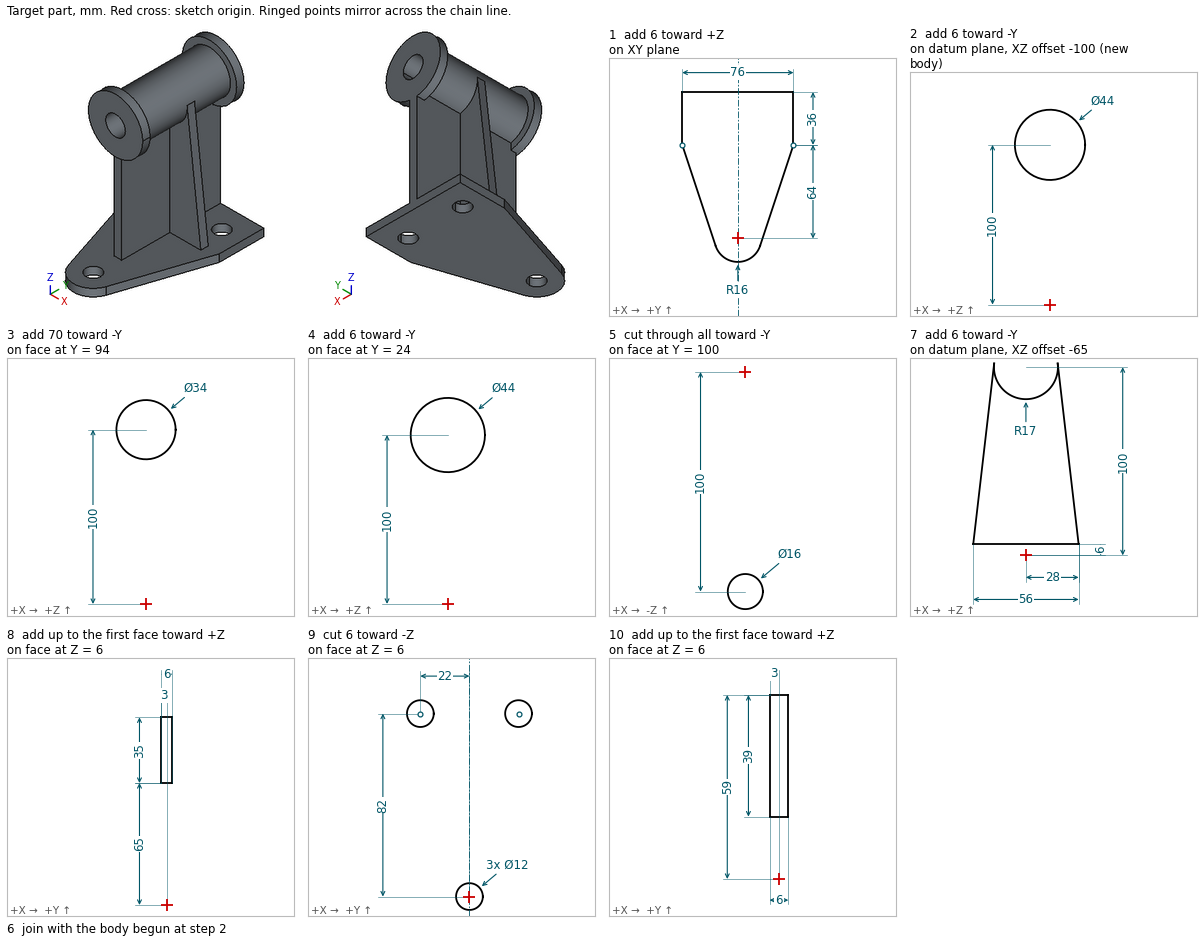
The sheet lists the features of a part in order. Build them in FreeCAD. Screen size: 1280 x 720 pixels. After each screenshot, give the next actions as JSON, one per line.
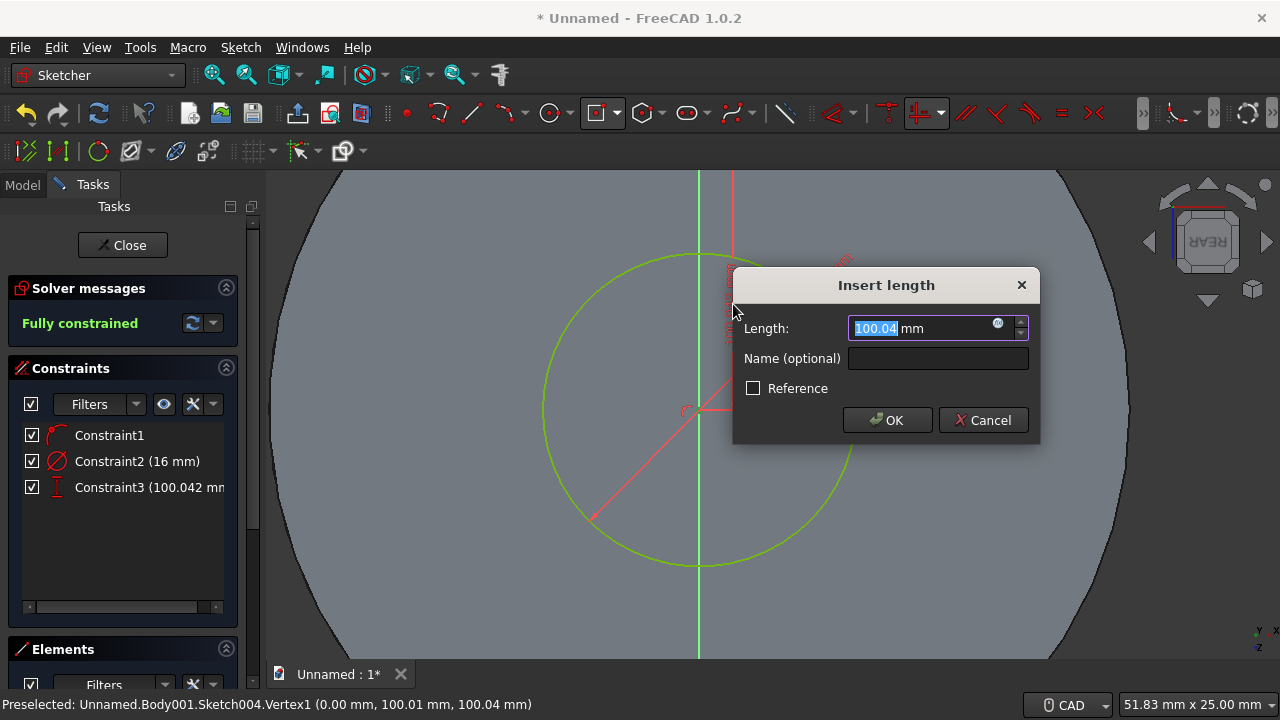
{"action": "type", "text": "100"}
{"action": "key", "text": "Return"}
{"action": "key", "text": "Escape"}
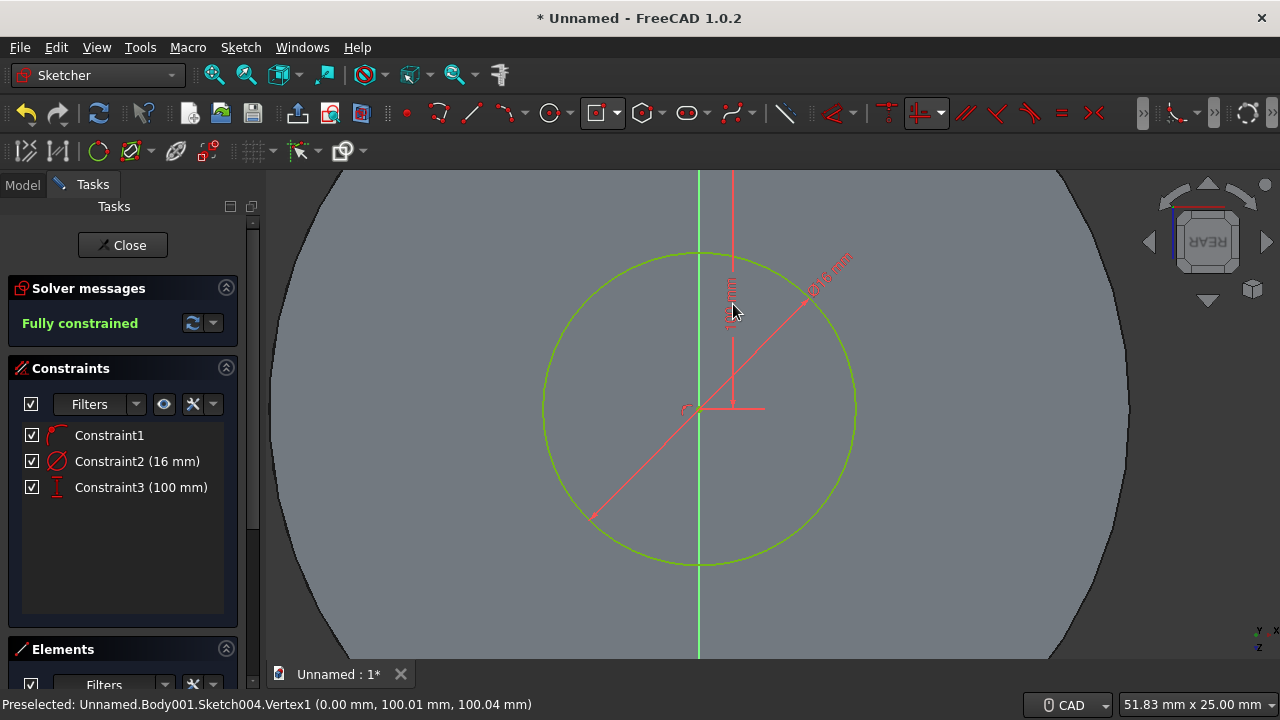
{"action": "left_click", "coordinate": [123, 245]}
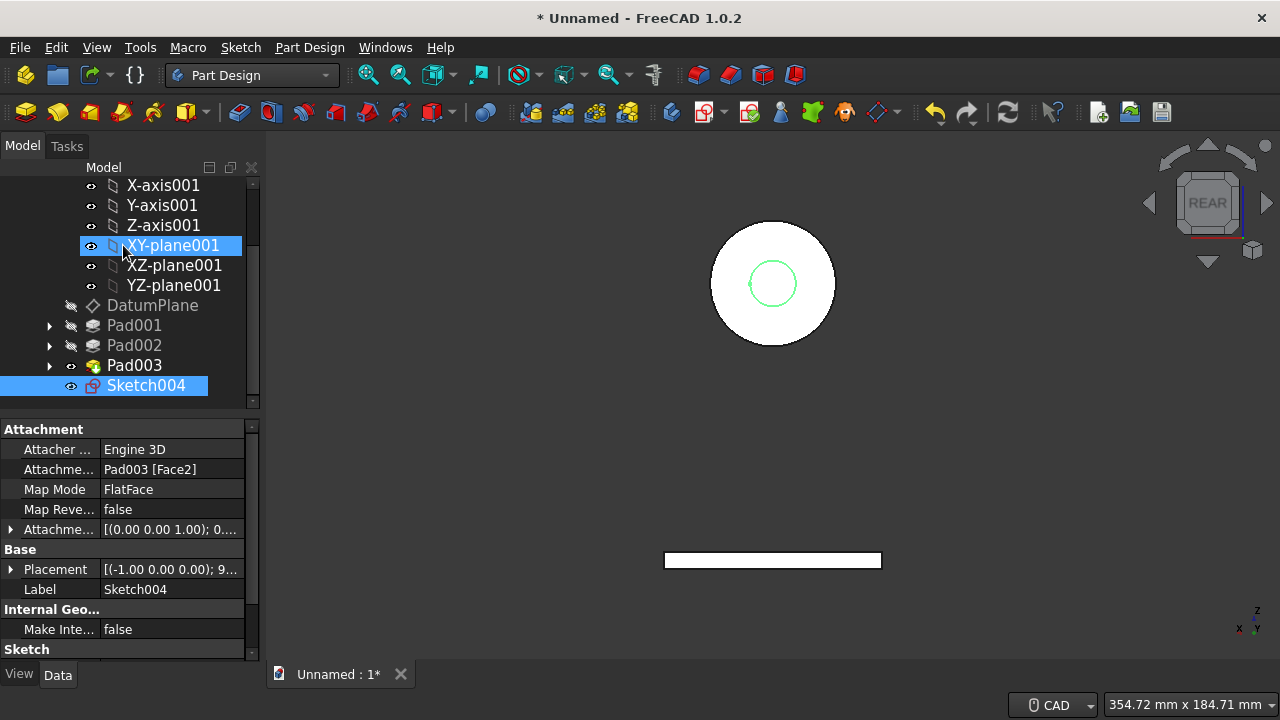
{"action": "left_click", "coordinate": [240, 112]}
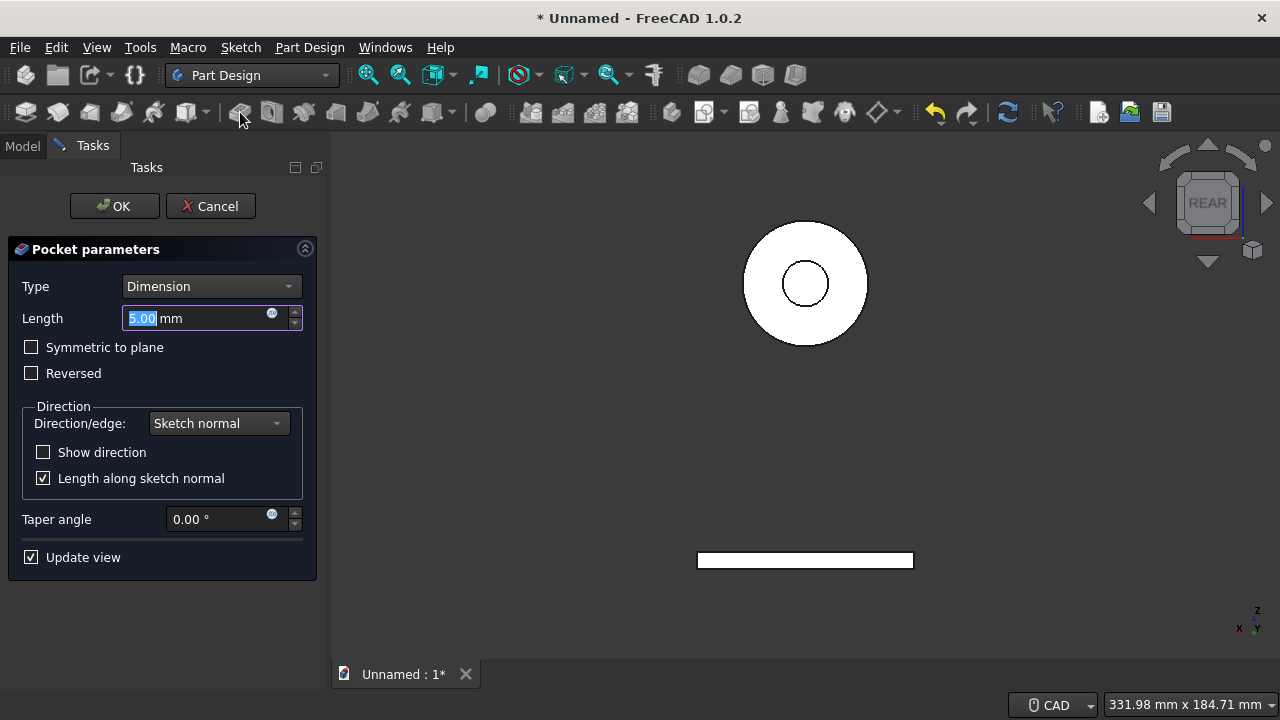
{"action": "left_click", "coordinate": [212, 286]}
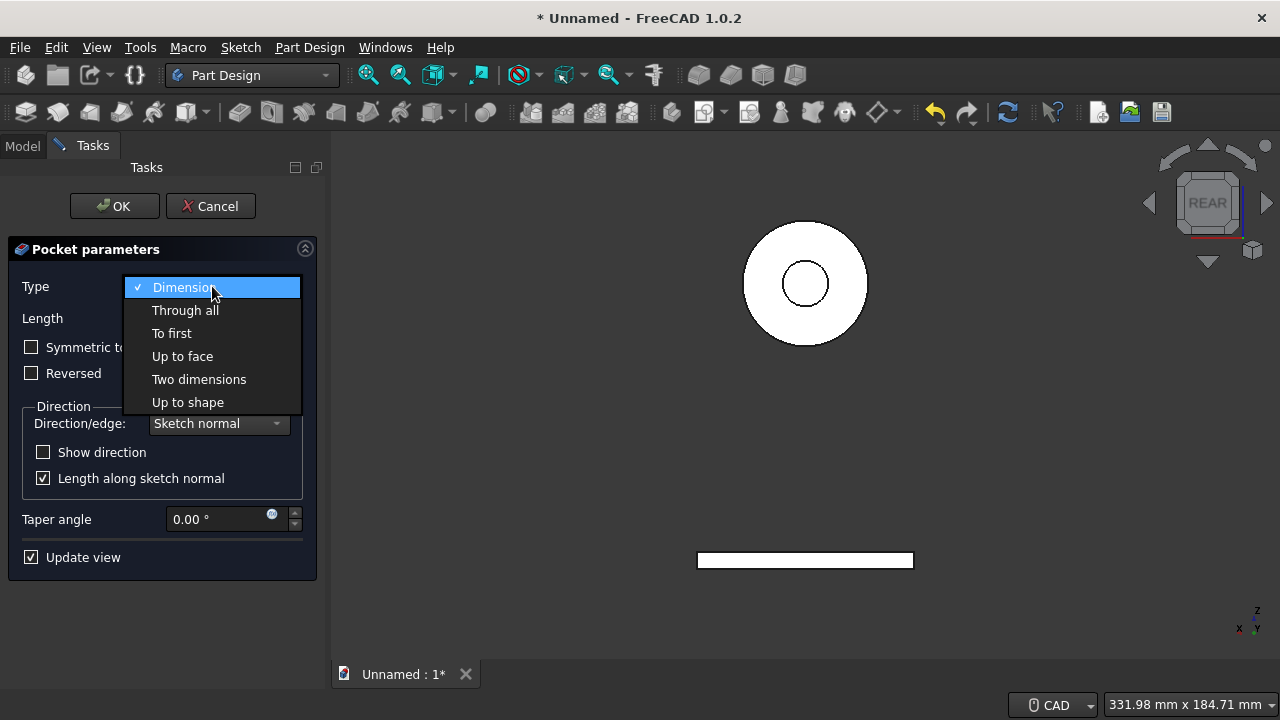
{"action": "left_click", "coordinate": [212, 310]}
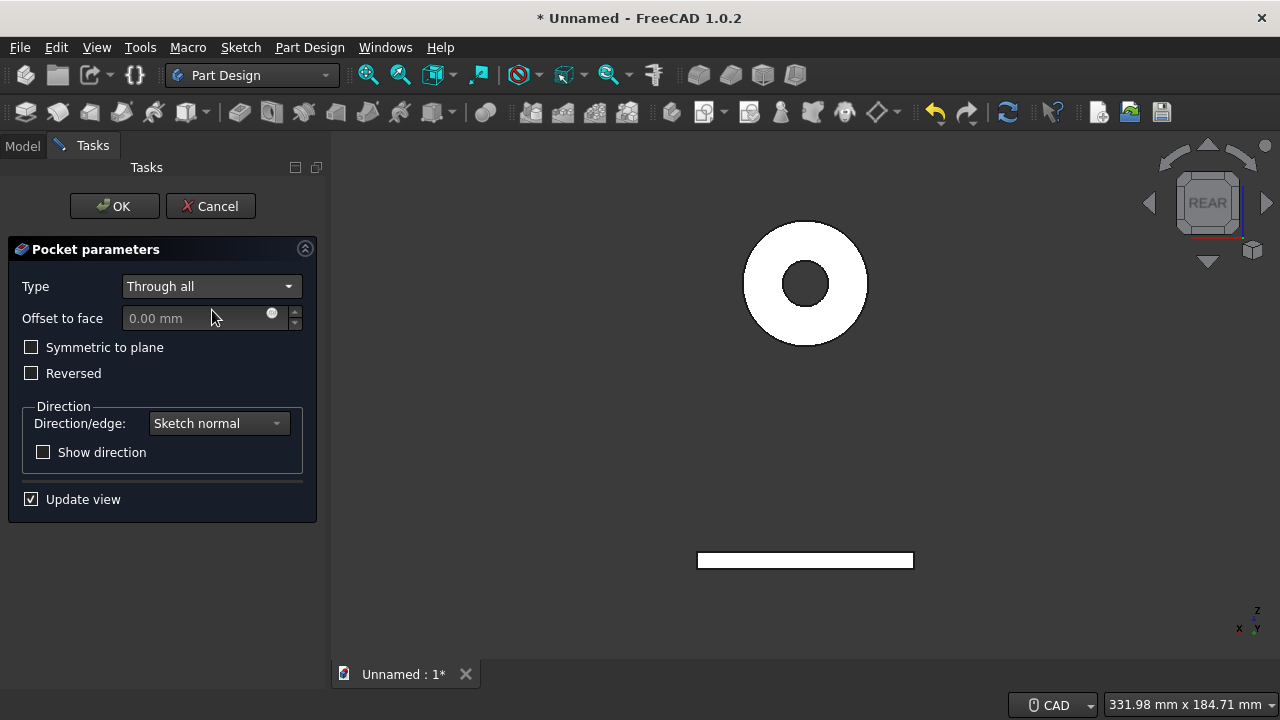
{"action": "left_click", "coordinate": [115, 206]}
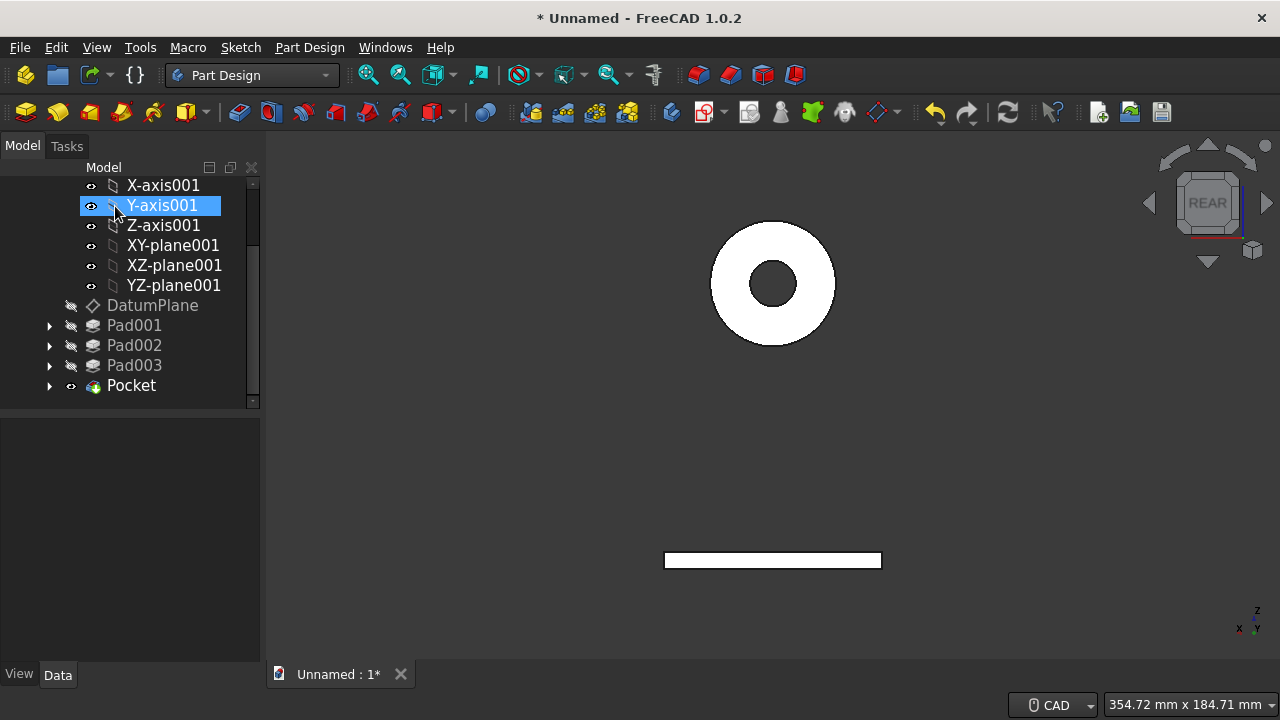
{"action": "key", "text": "v f"}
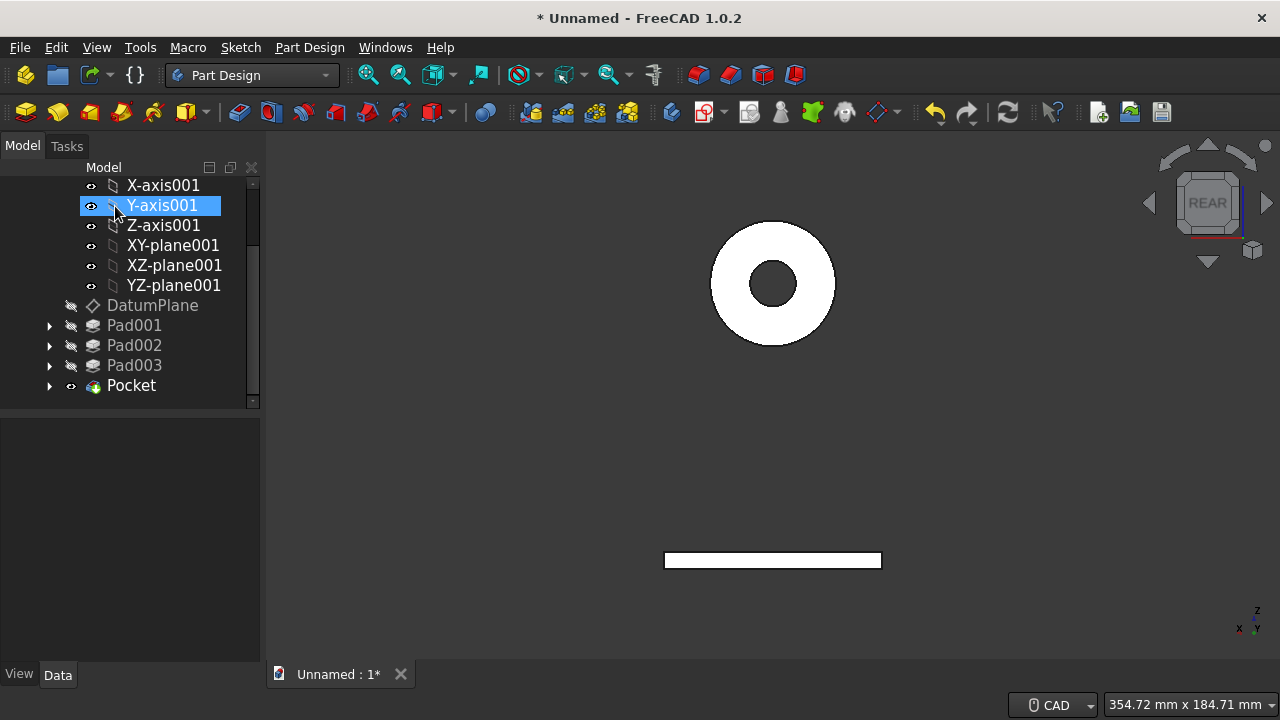
{"action": "scroll", "coordinate": [160, 281], "scroll_direction": "down", "scroll_amount": 3}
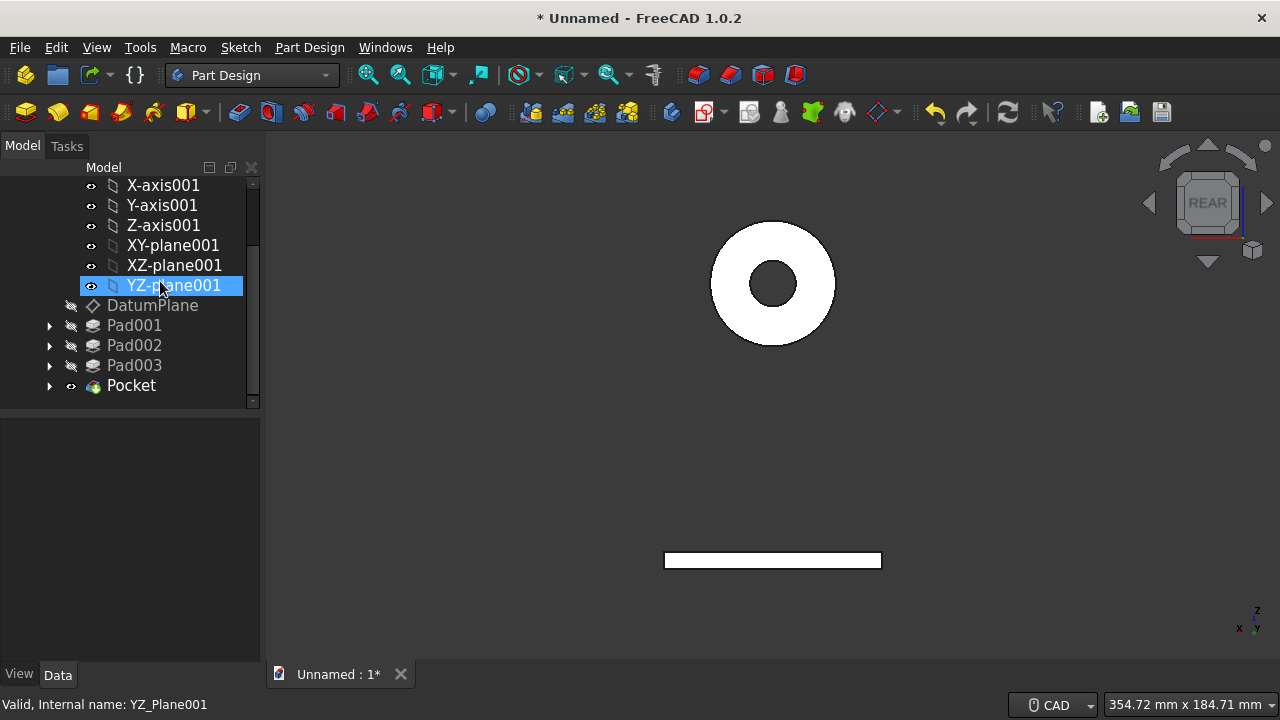
{"action": "scroll", "coordinate": [160, 281], "scroll_direction": "up", "scroll_amount": 15}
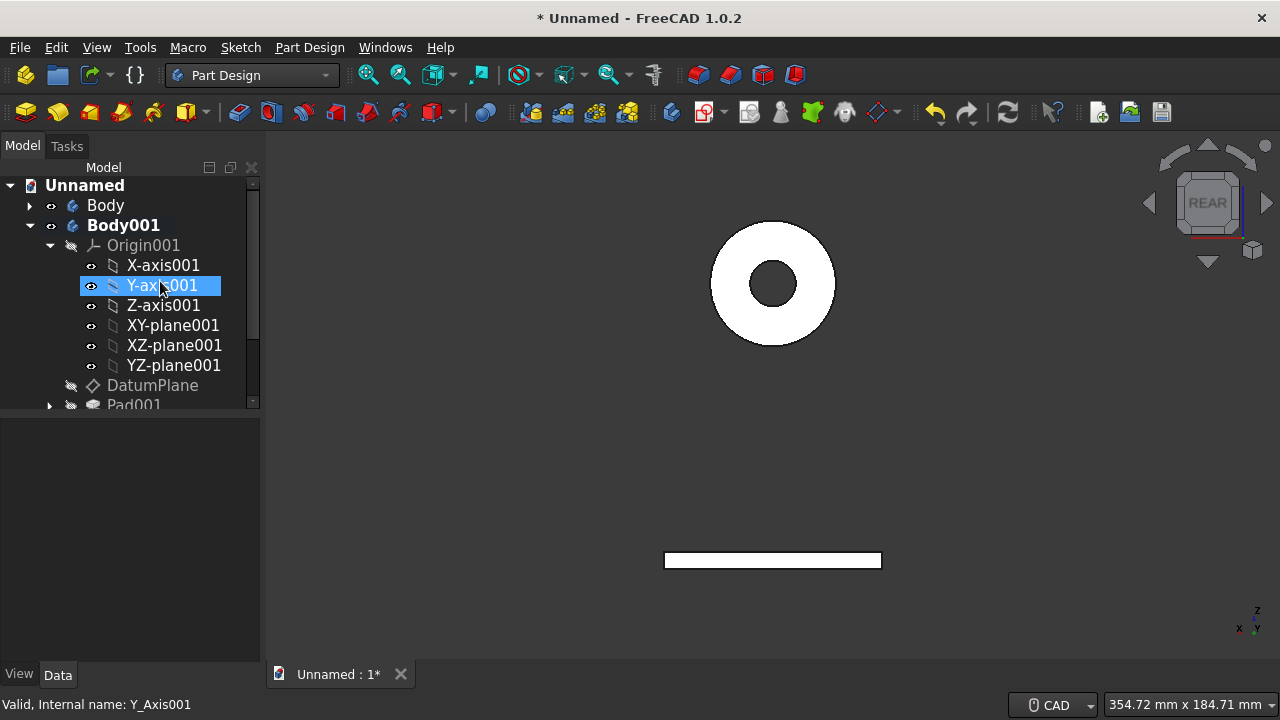
{"action": "double_click", "coordinate": [96, 206]}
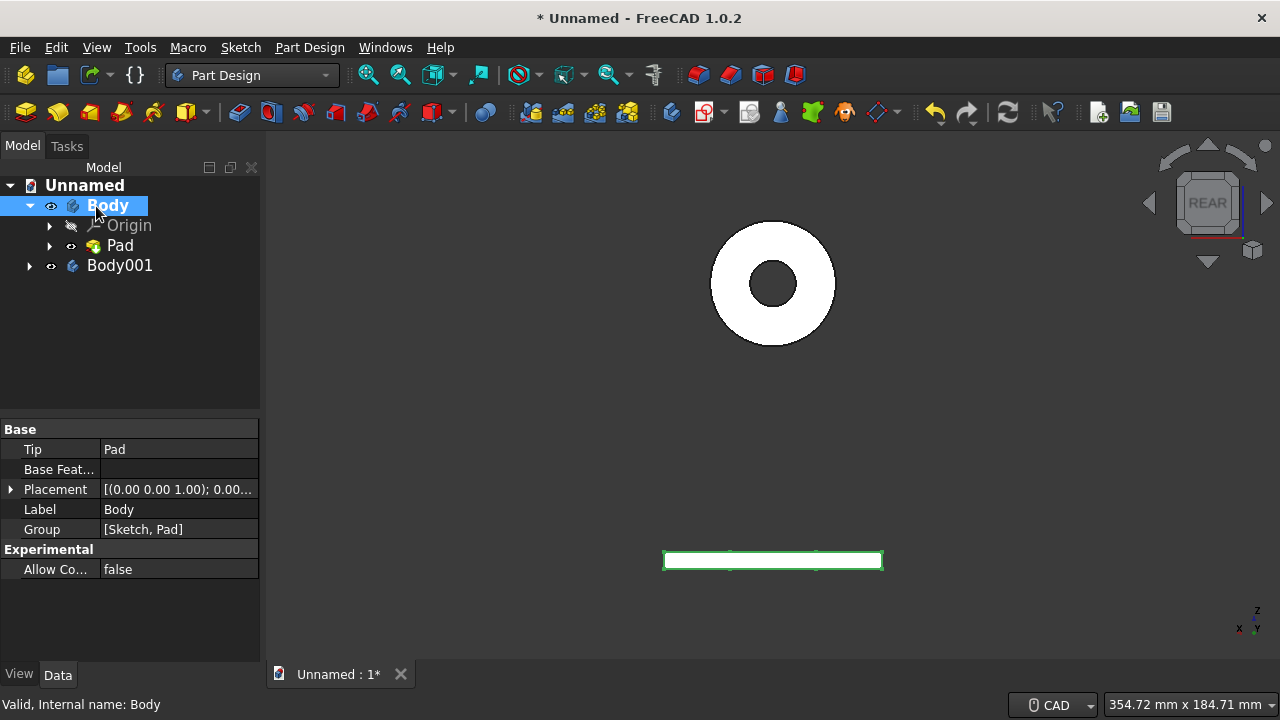
{"action": "left_click", "coordinate": [96, 206]}